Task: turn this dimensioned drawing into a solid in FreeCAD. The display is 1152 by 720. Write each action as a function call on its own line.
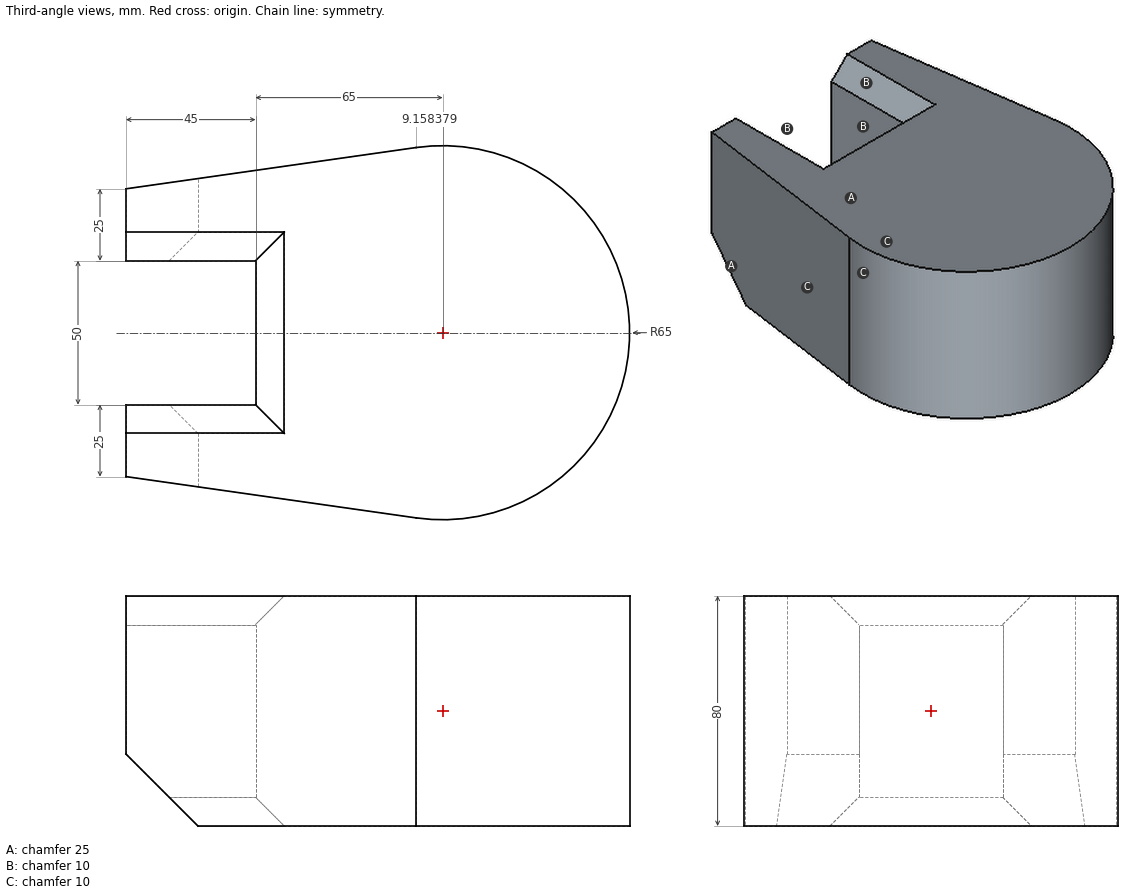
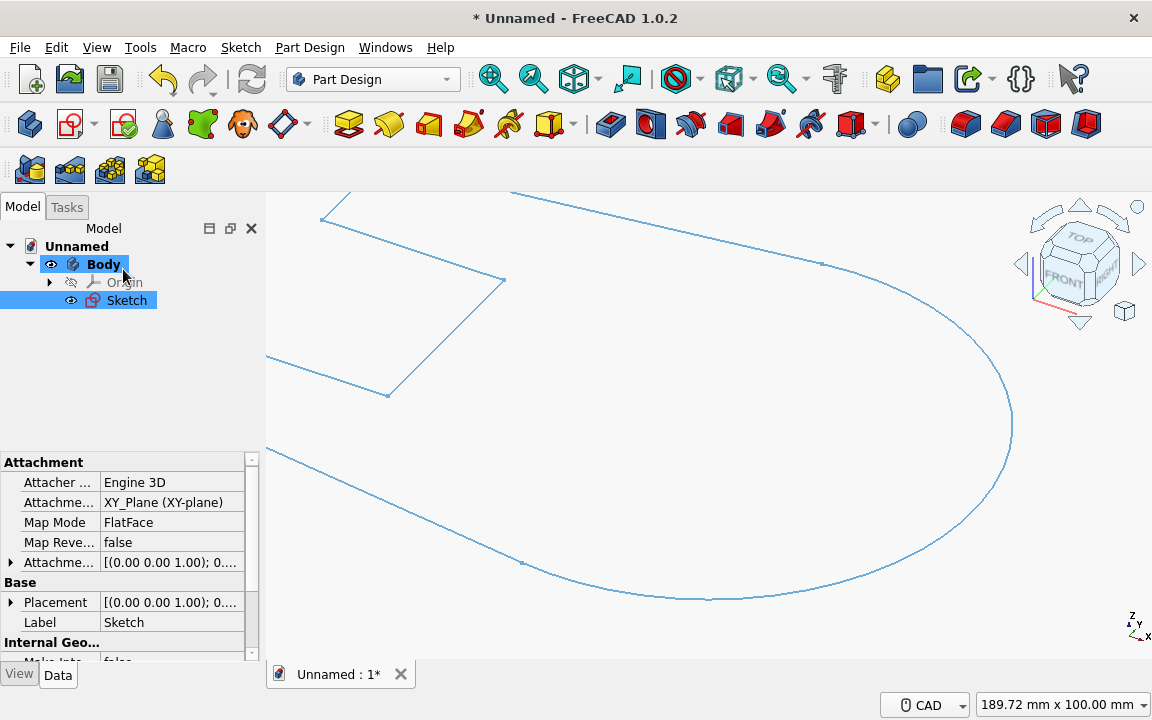
click(350, 124)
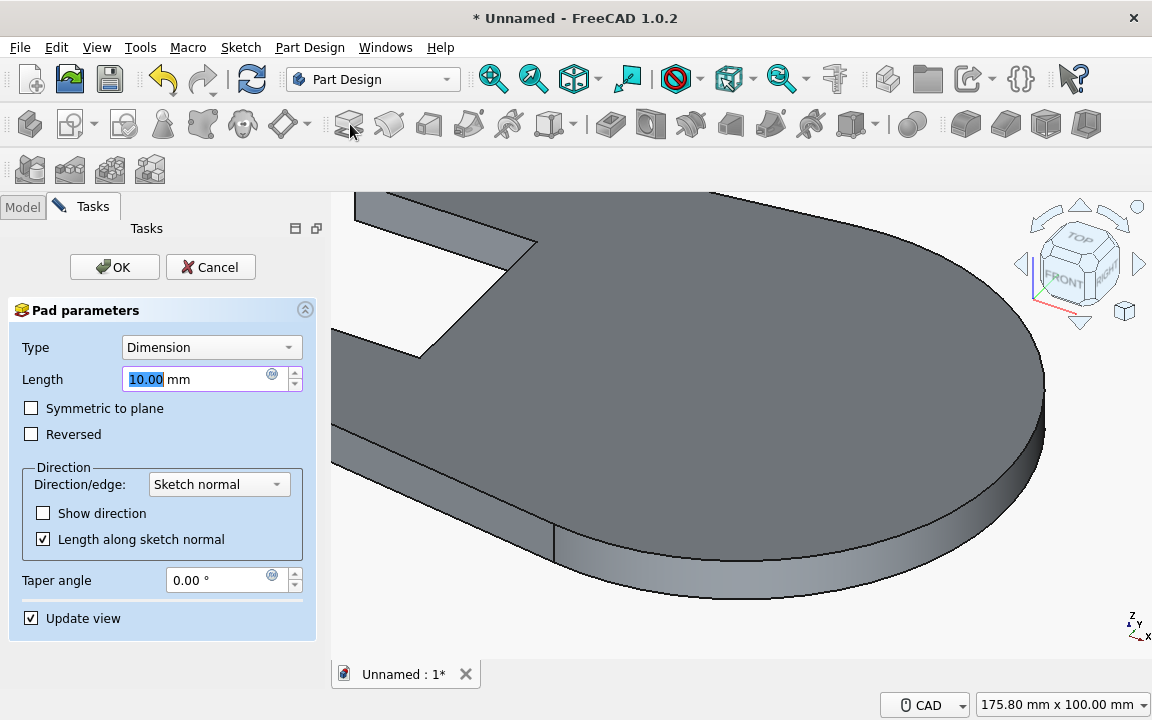
text(80)
key(Tab)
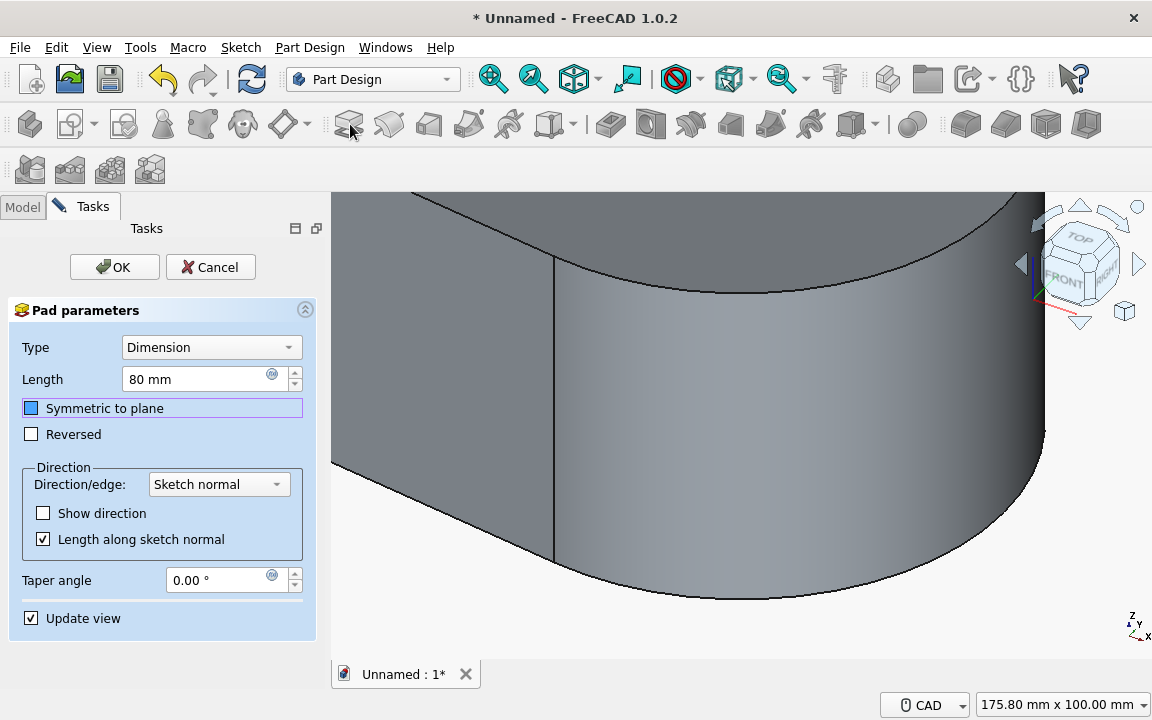
click(30, 408)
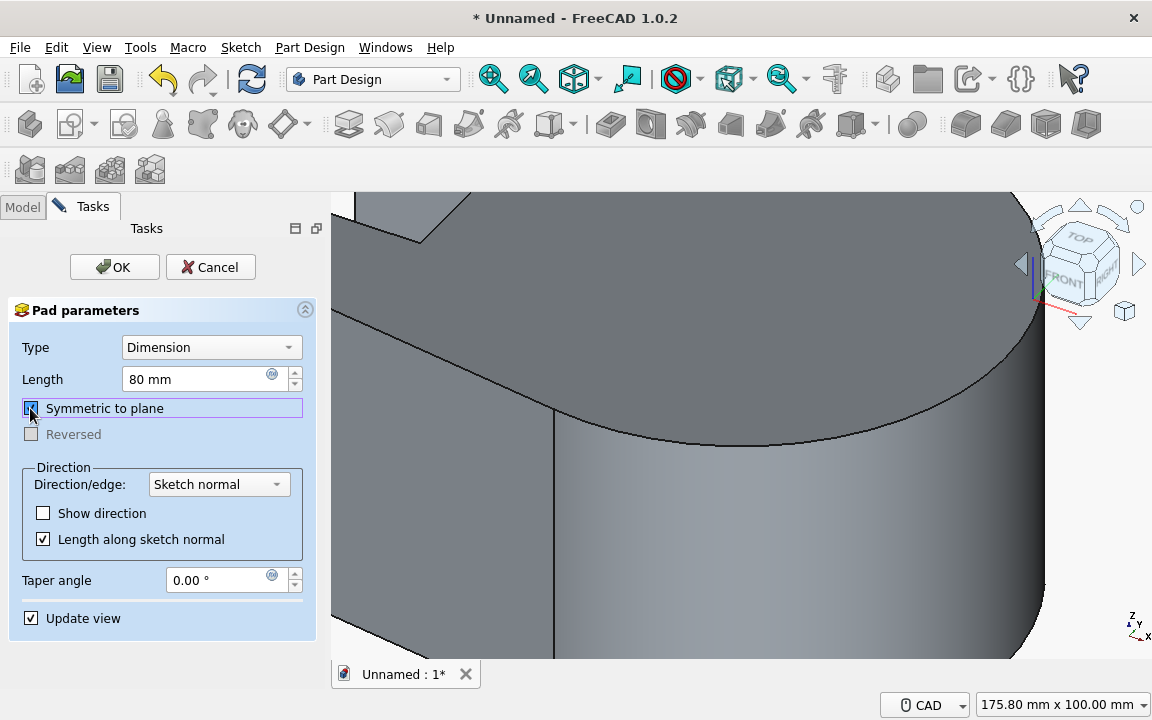
click(115, 267)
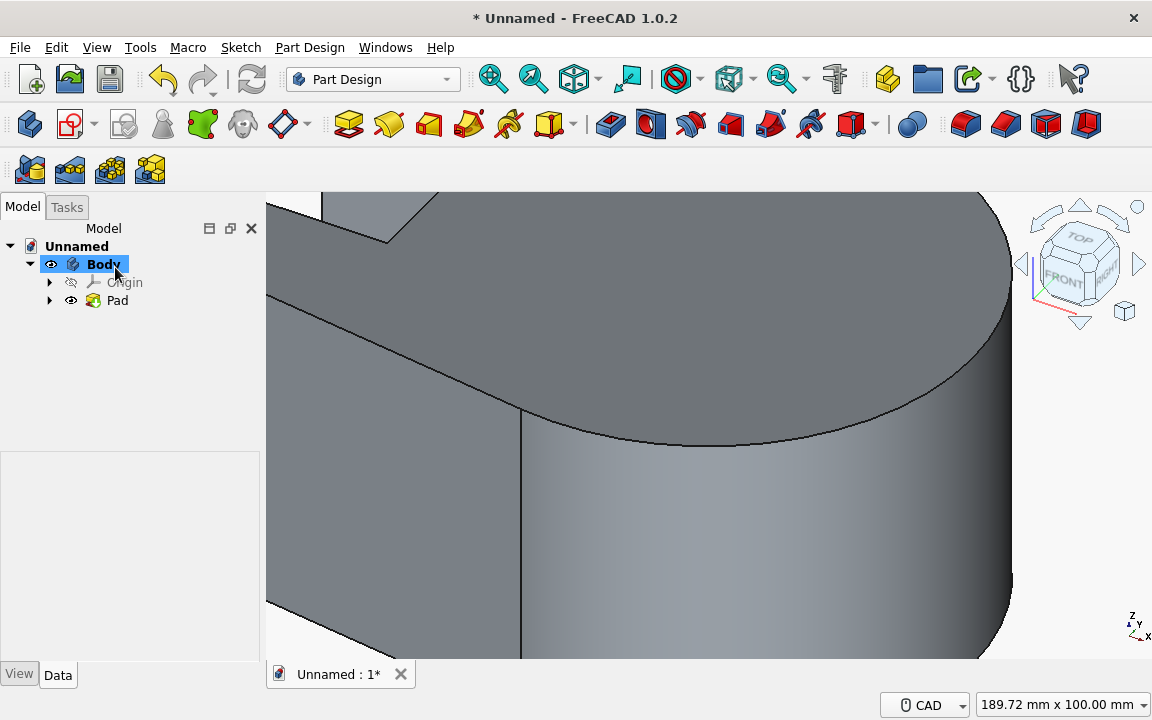
click(494, 80)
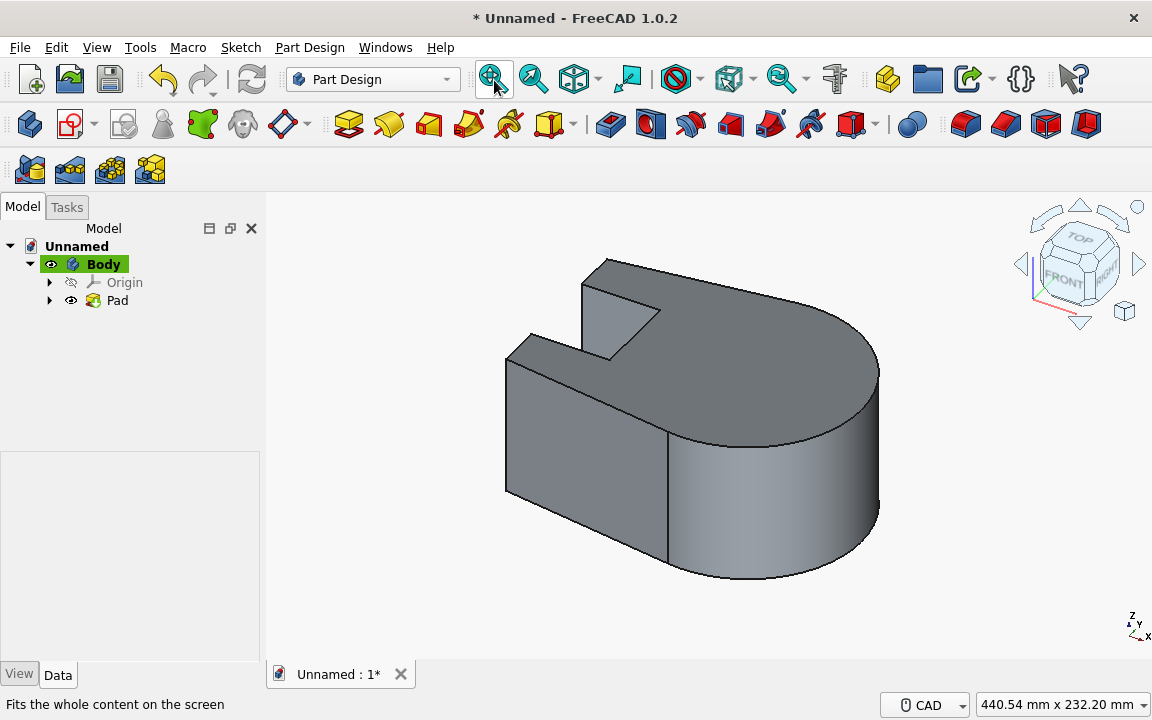
key(0)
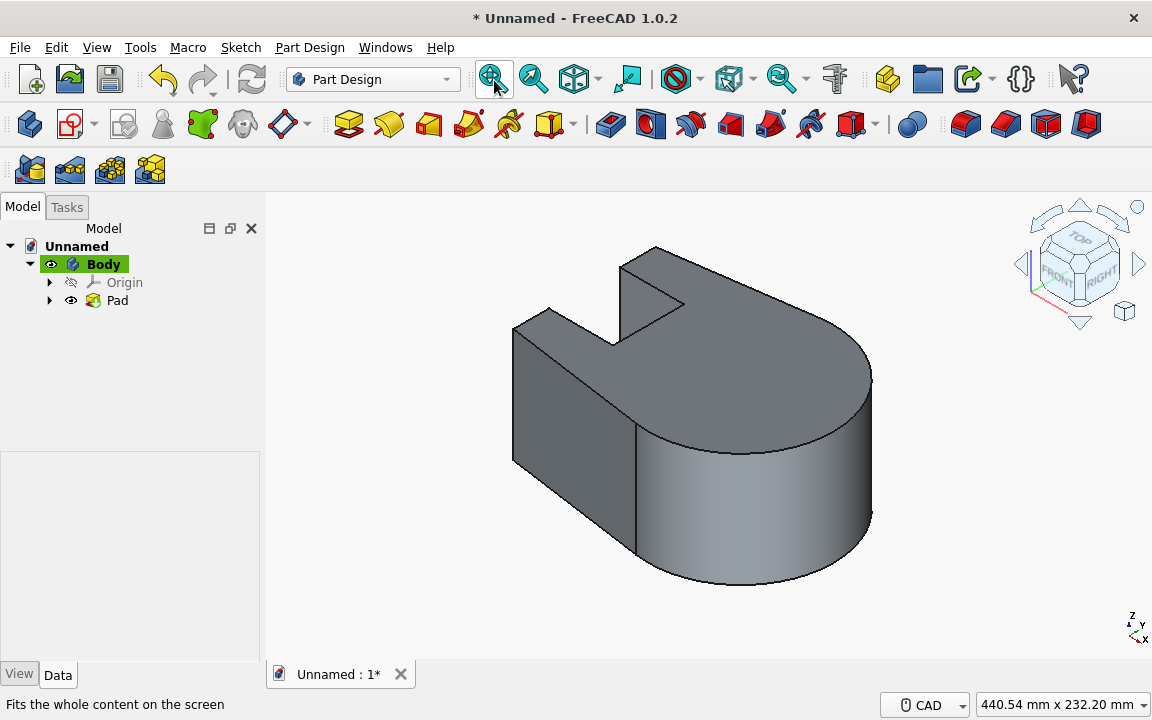
key(2)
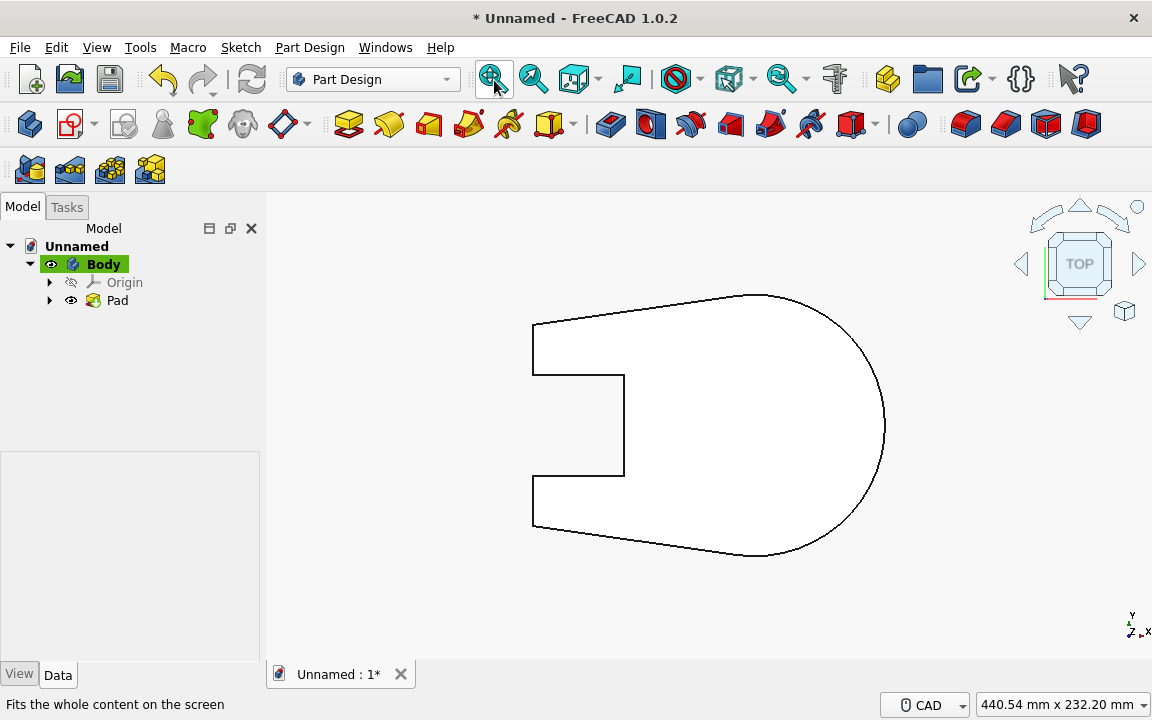
key(1)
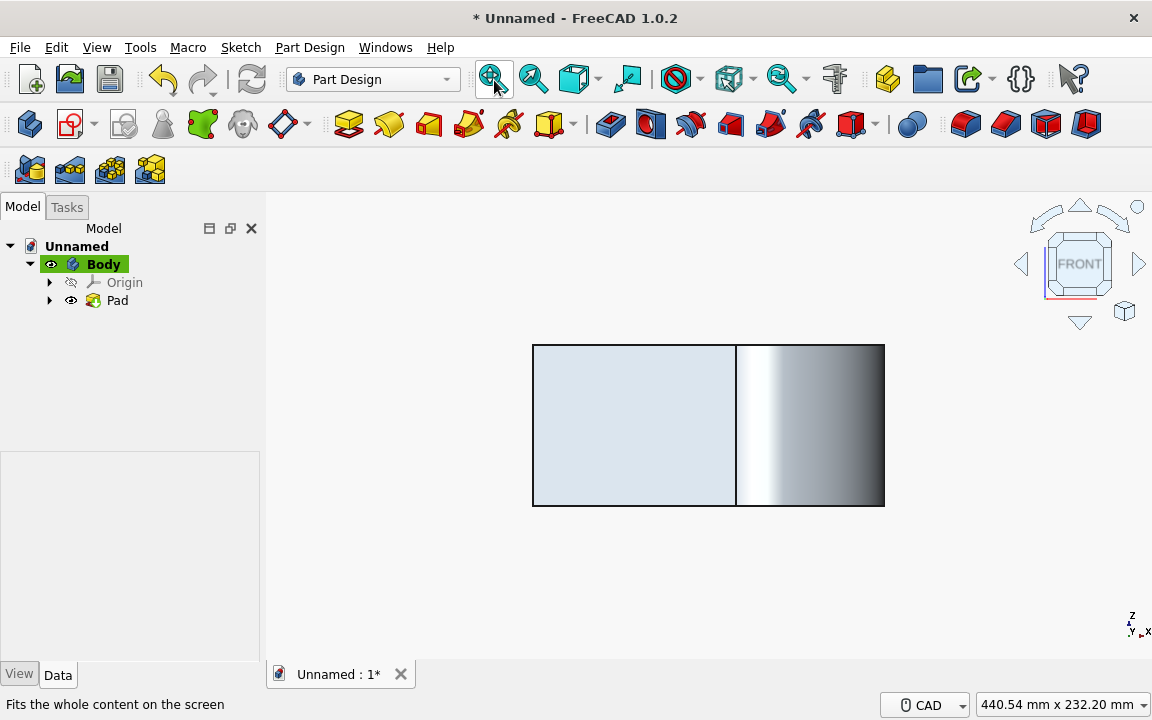
click(494, 80)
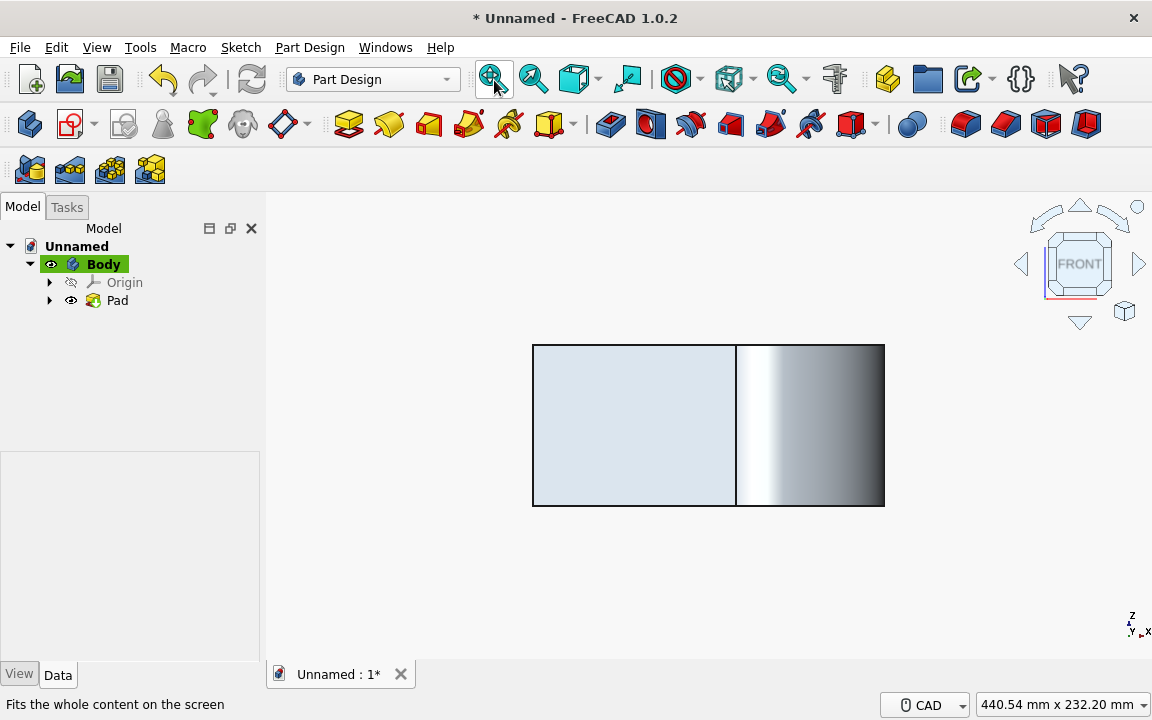
key(3)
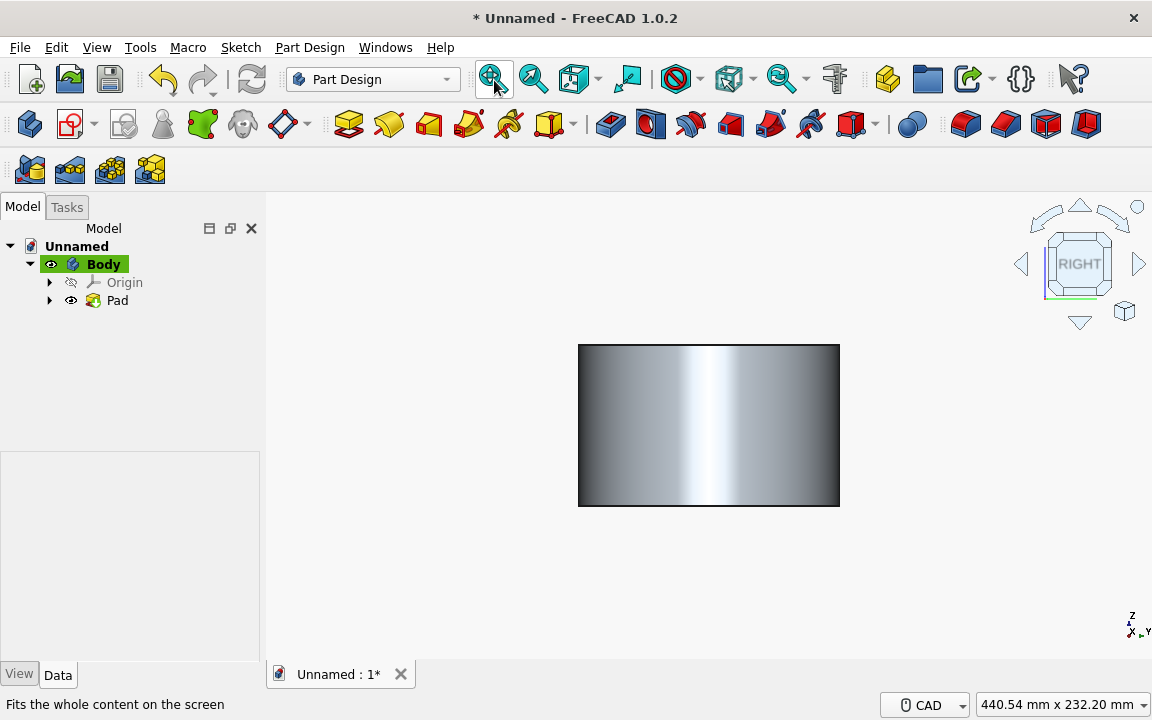
click(494, 80)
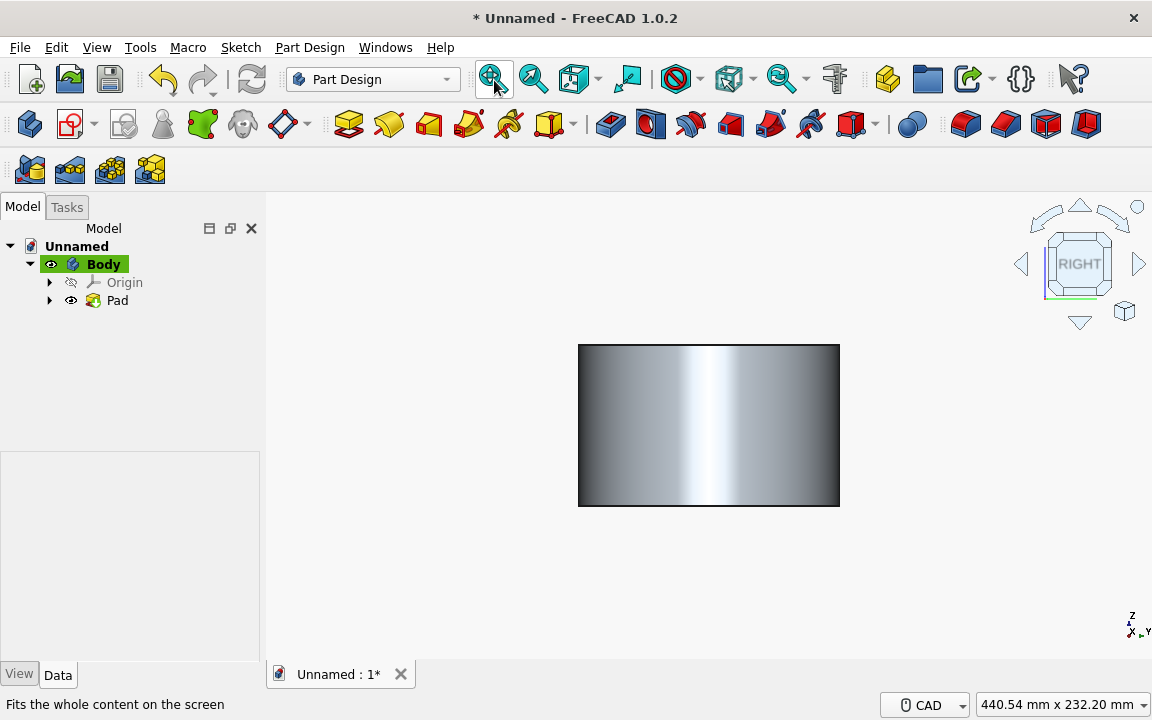
key(5)